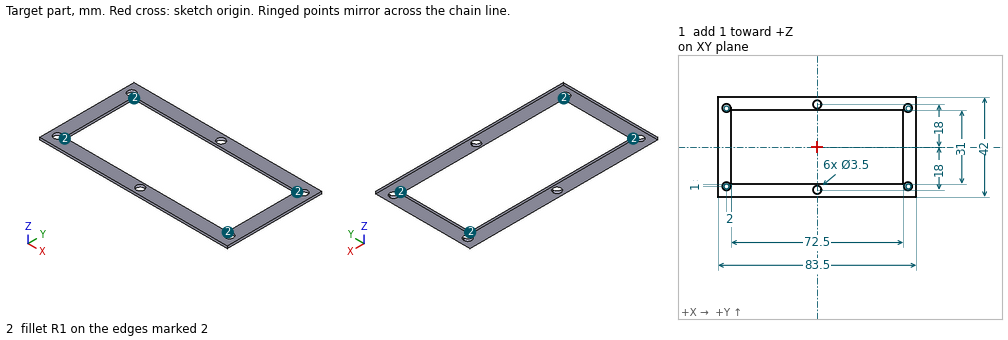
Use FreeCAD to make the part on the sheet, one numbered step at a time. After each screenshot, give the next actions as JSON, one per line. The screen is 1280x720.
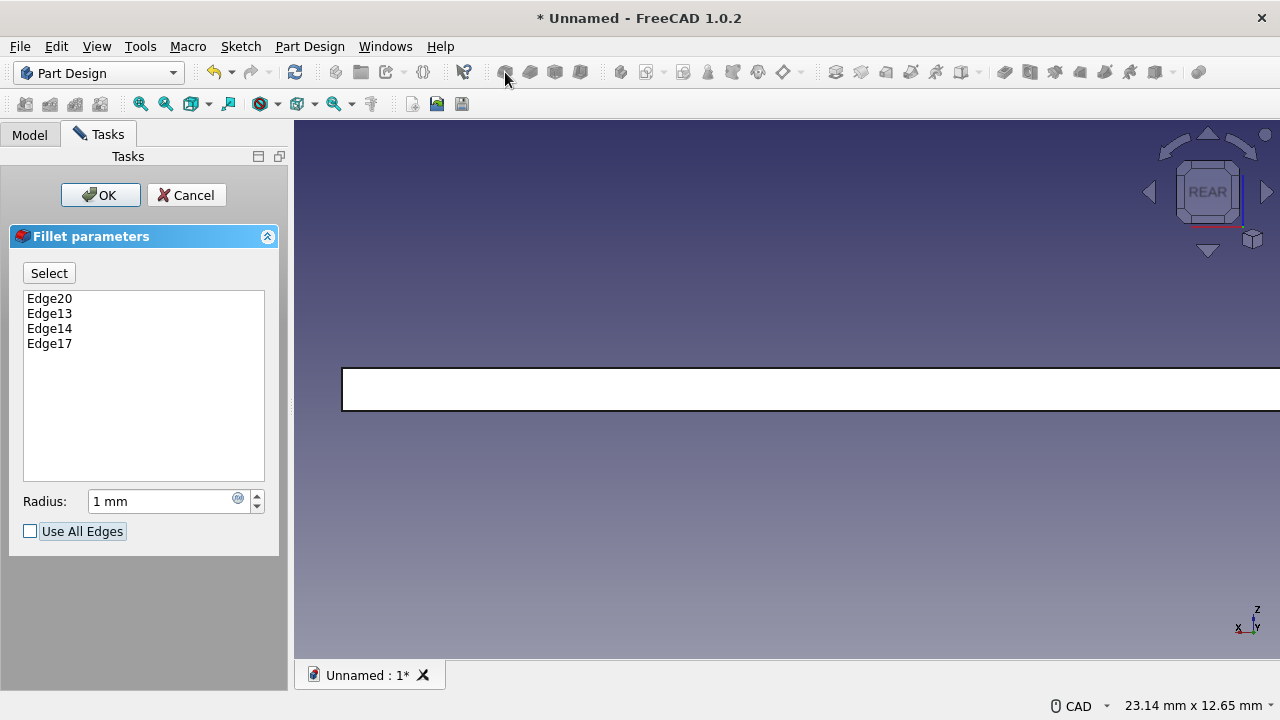
{"action": "left_click", "coordinate": [101, 195]}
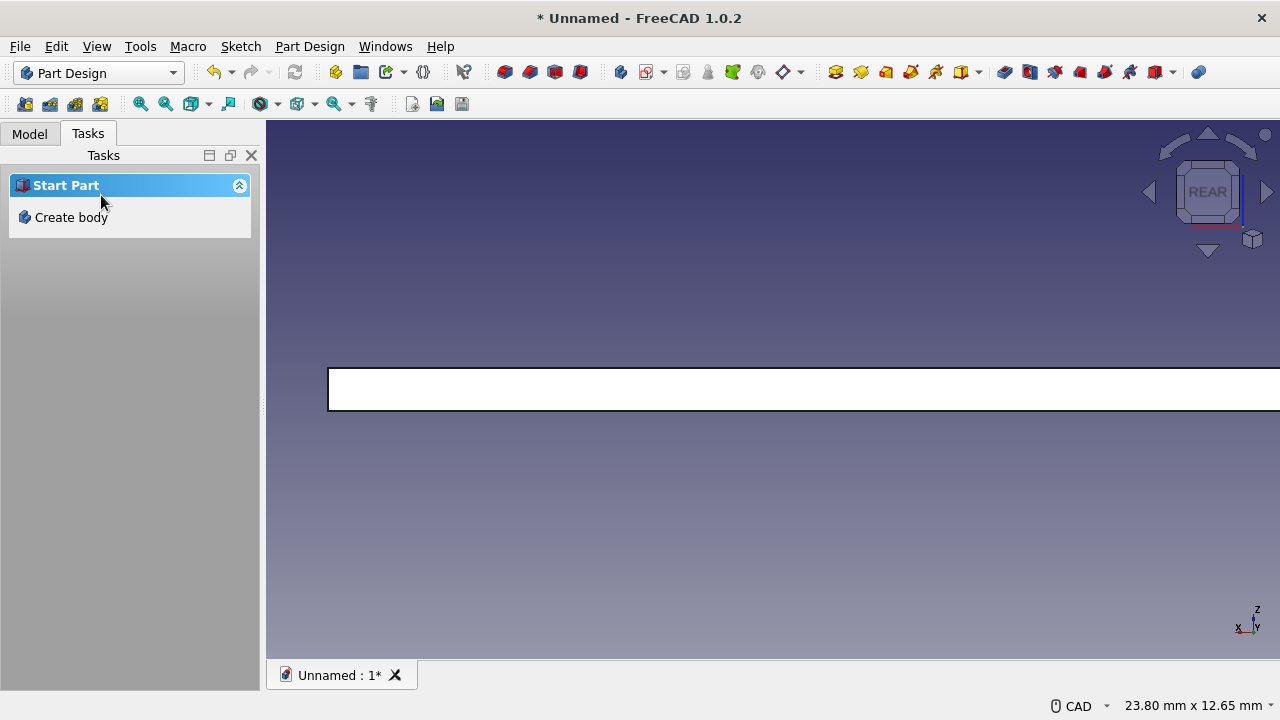
{"action": "key", "text": "0"}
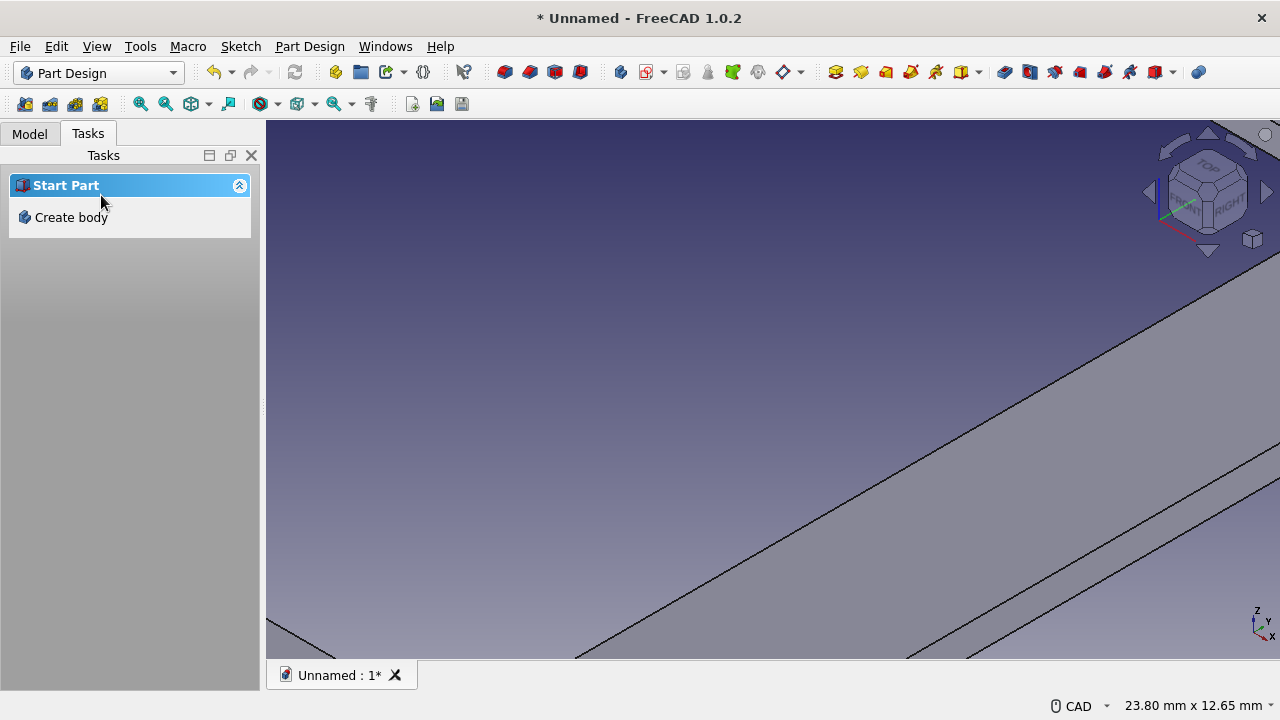
{"action": "key", "text": "v f"}